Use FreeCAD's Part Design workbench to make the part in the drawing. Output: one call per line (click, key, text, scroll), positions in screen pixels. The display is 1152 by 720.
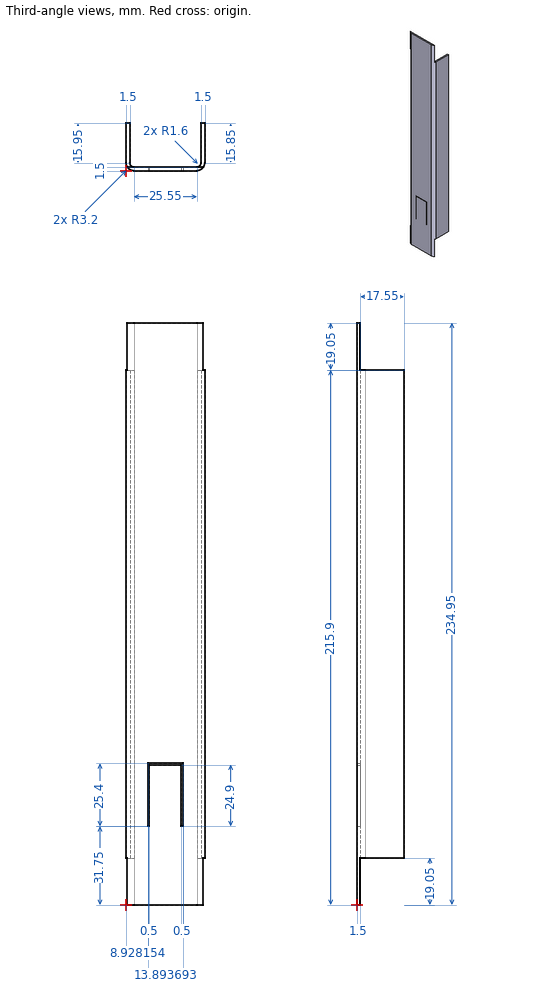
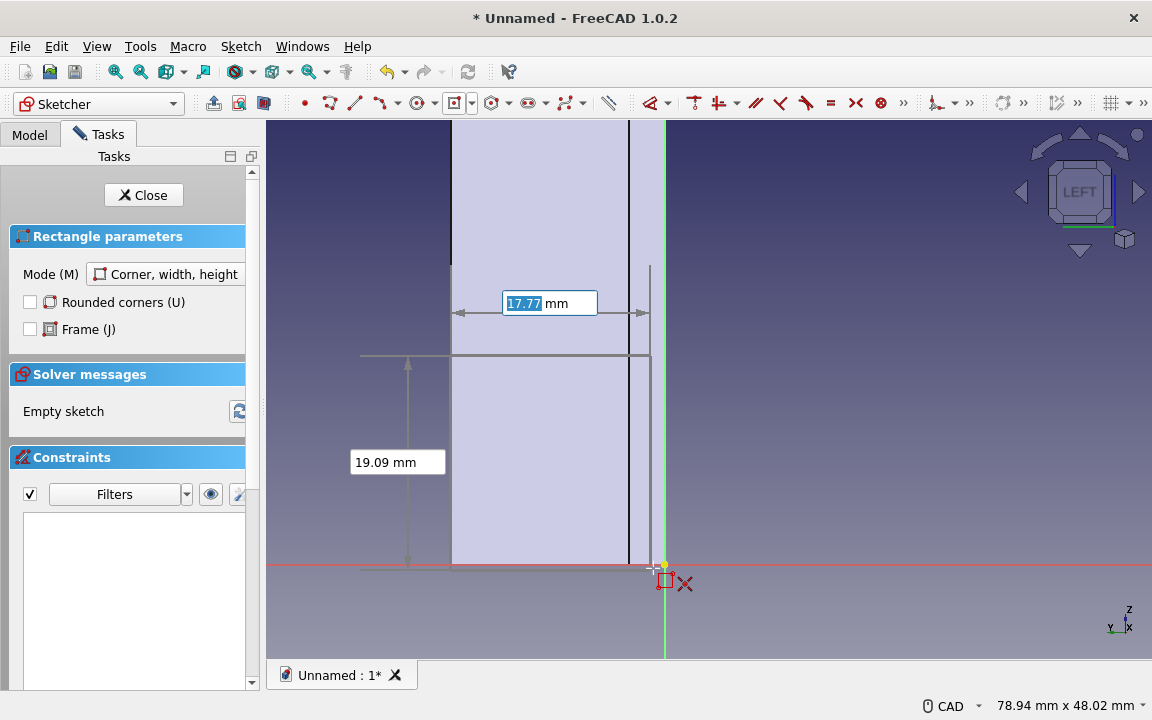
click(648, 565)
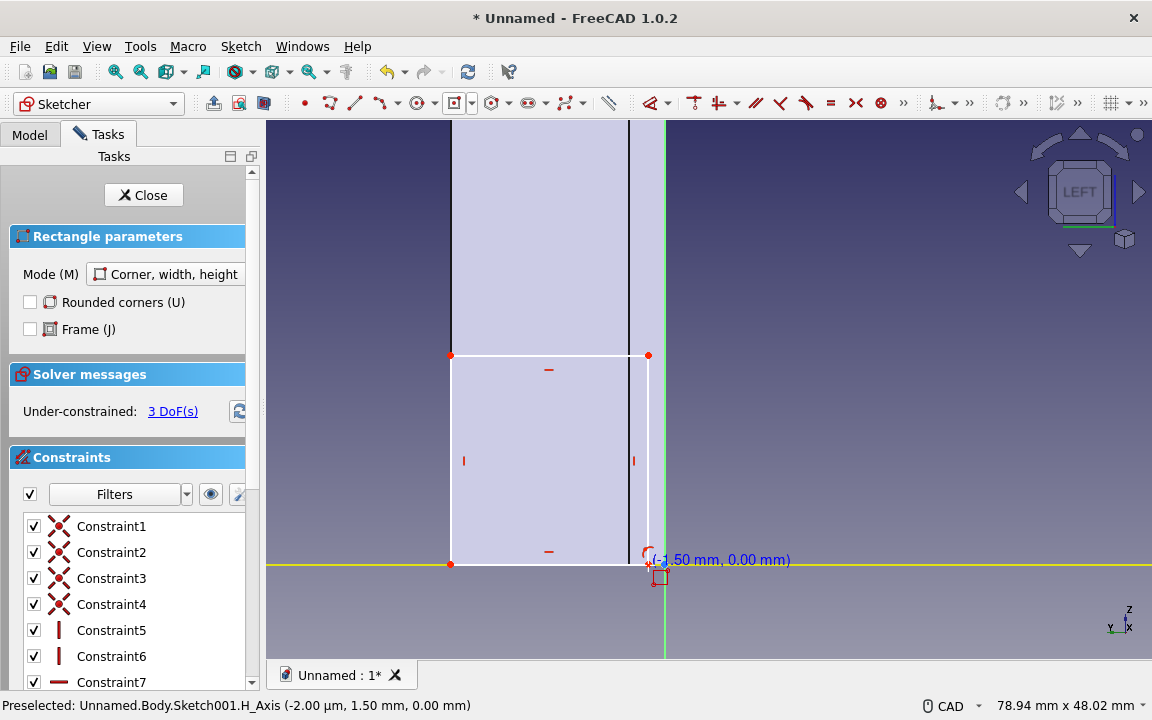
scroll(653, 568, down, 10)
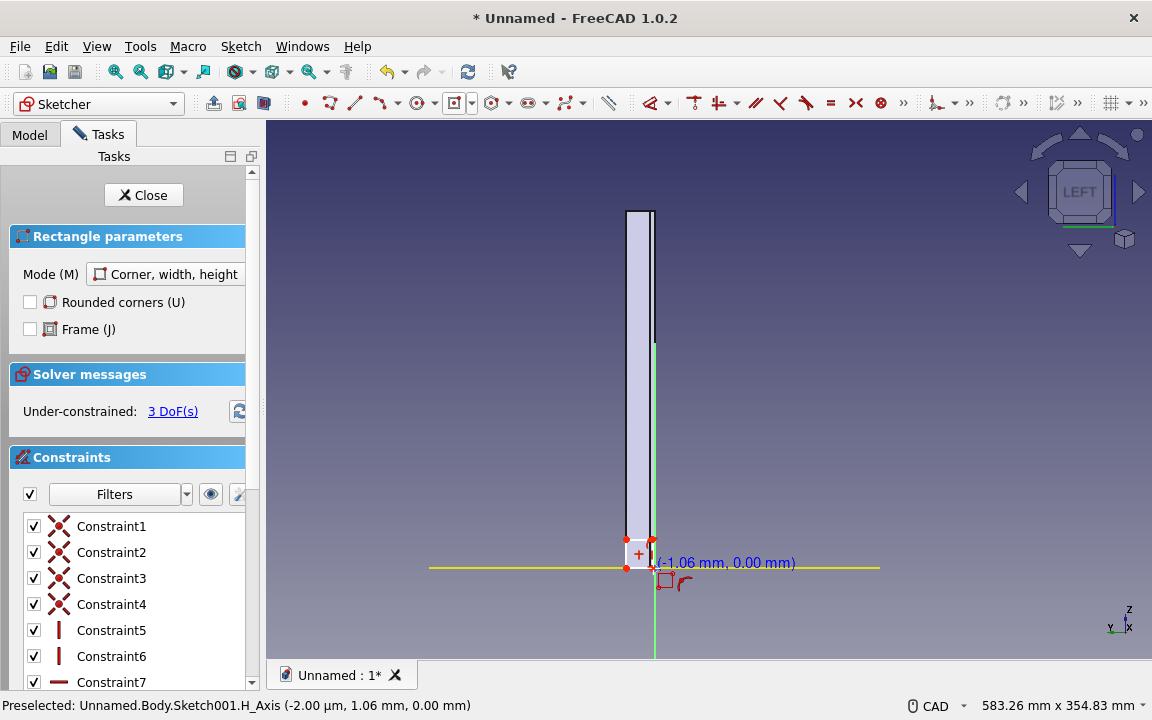
click(626, 211)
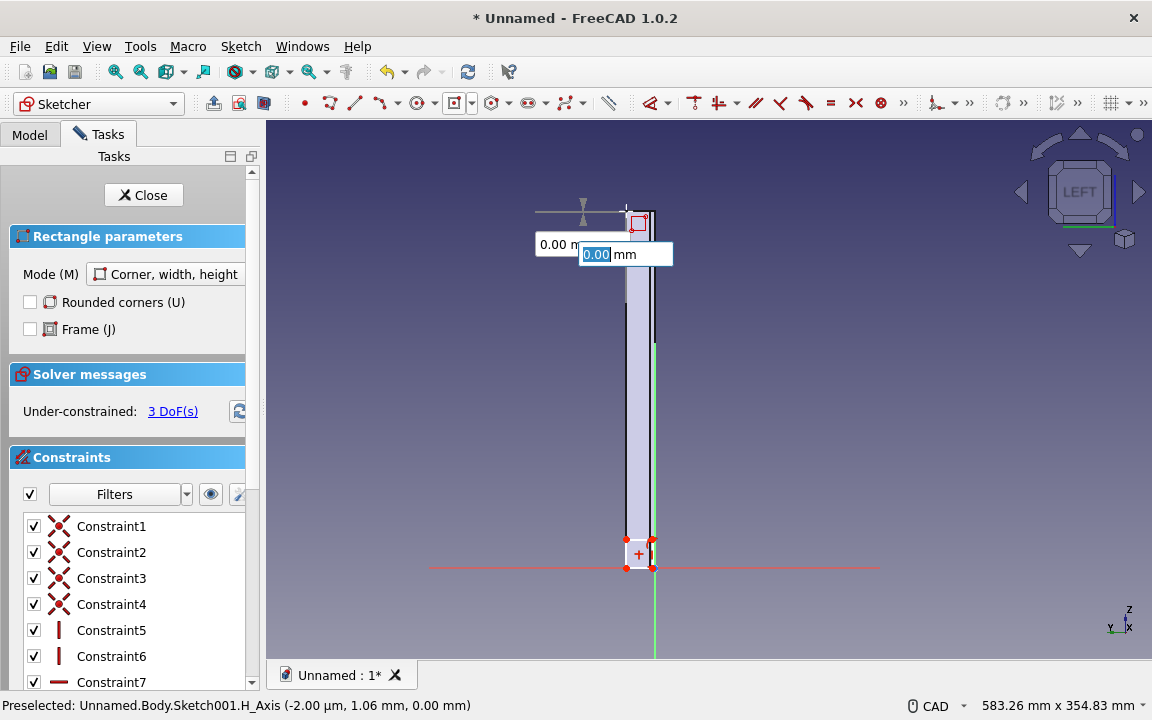
scroll(653, 240, up, 10)
move(648, 241)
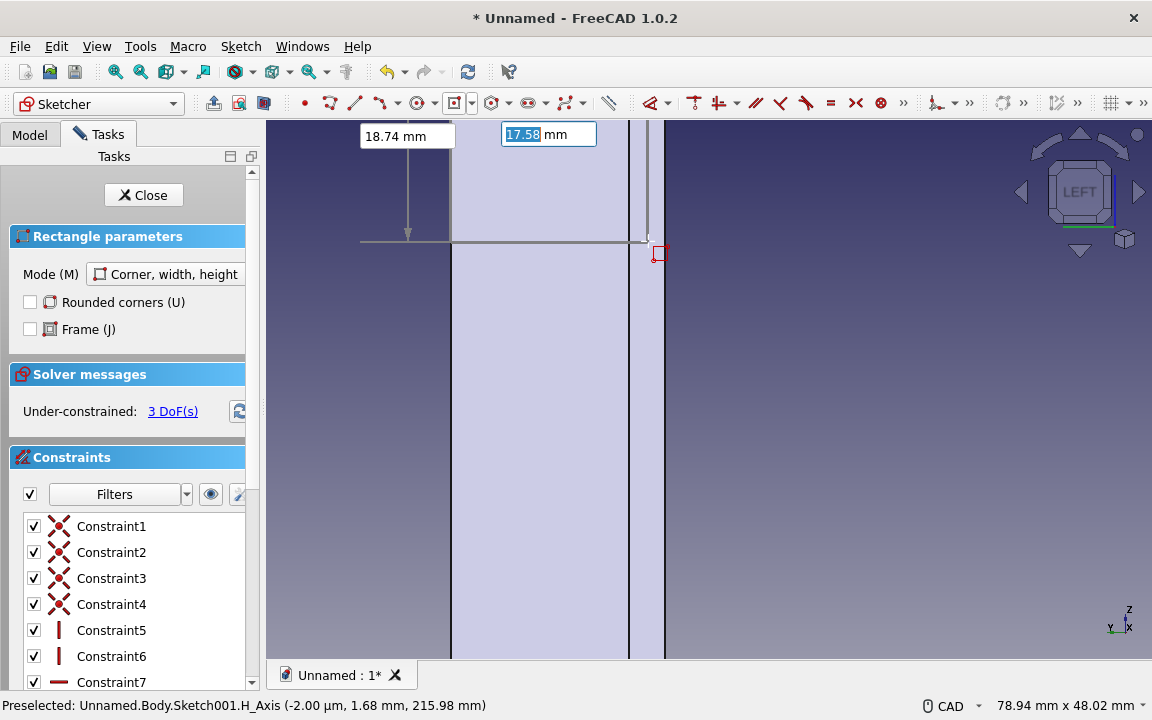
text(17.55)
key(Tab)
text(19.05)
key(Return)
key(Escape)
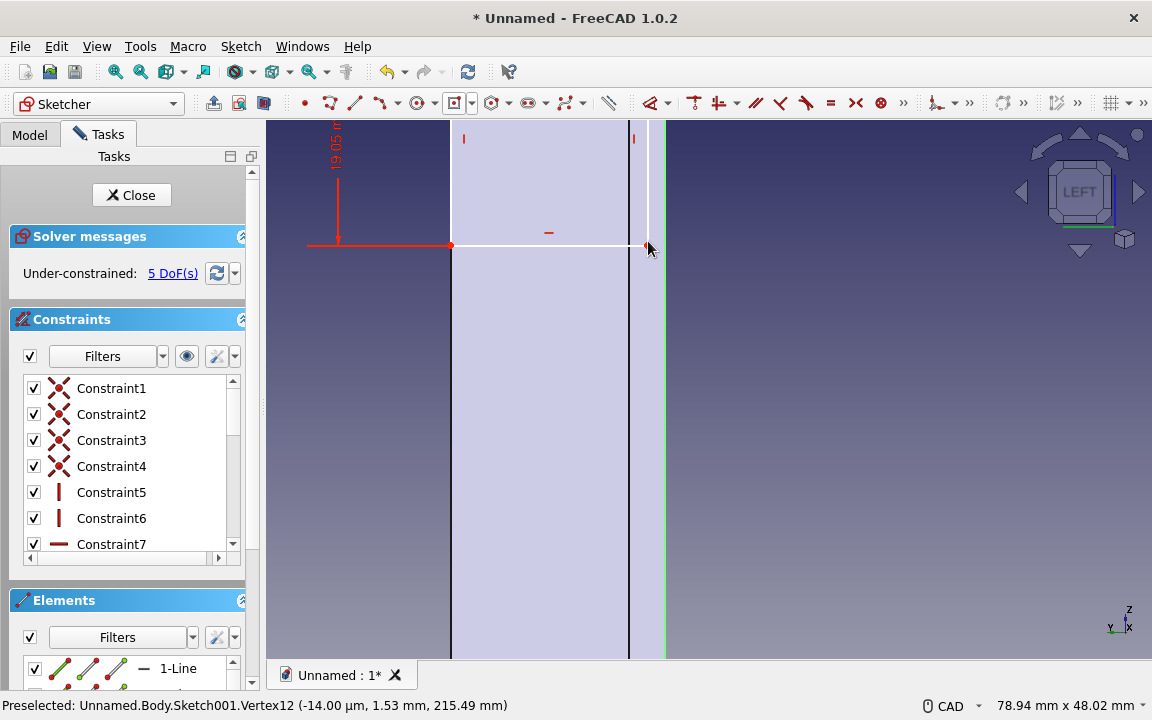
click(650, 104)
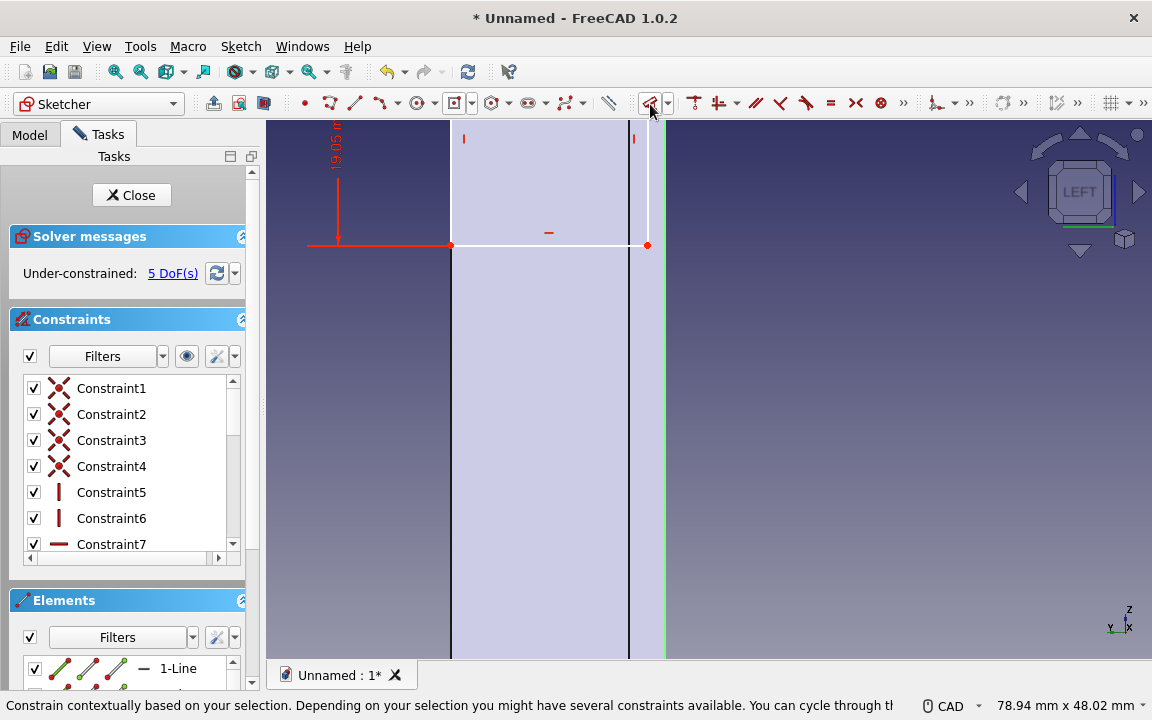
scroll(653, 240, down, 10)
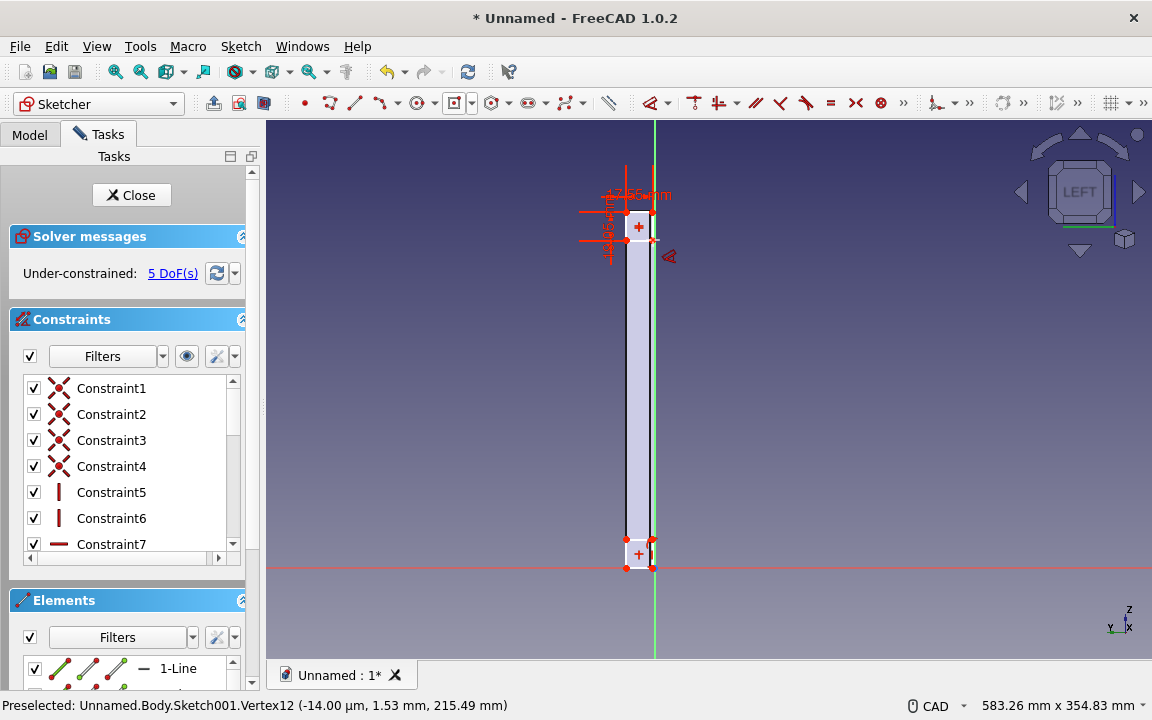
scroll(653, 568, up, 15)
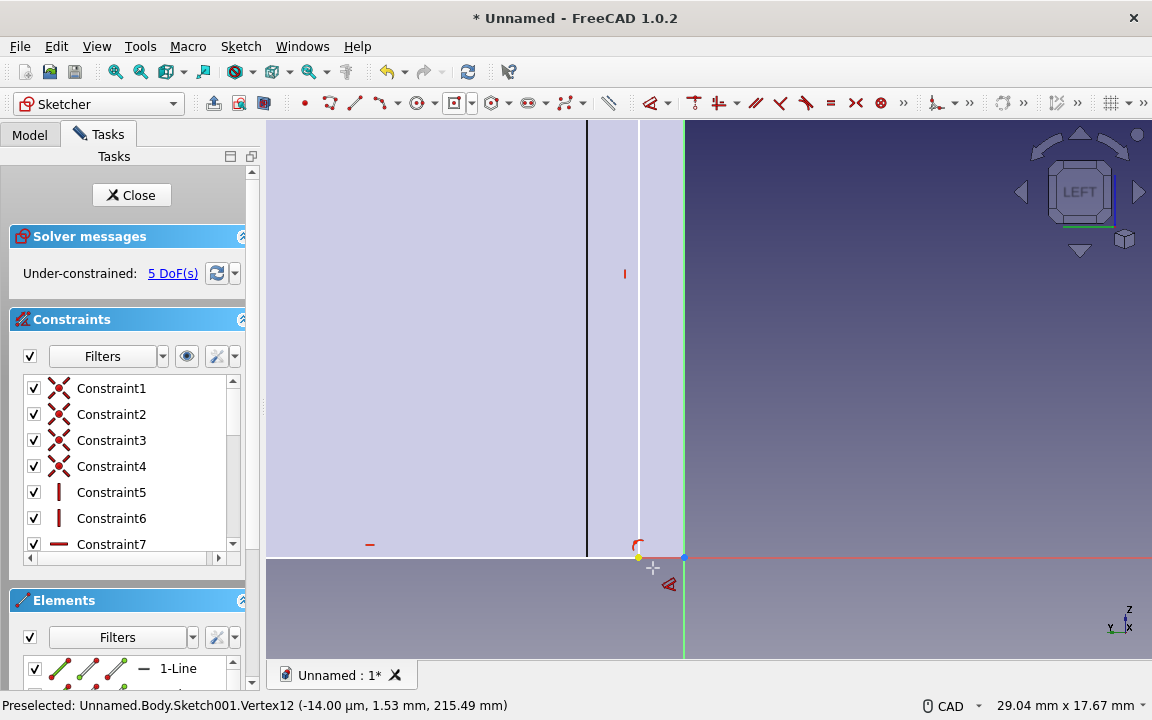
click(639, 558)
click(662, 592)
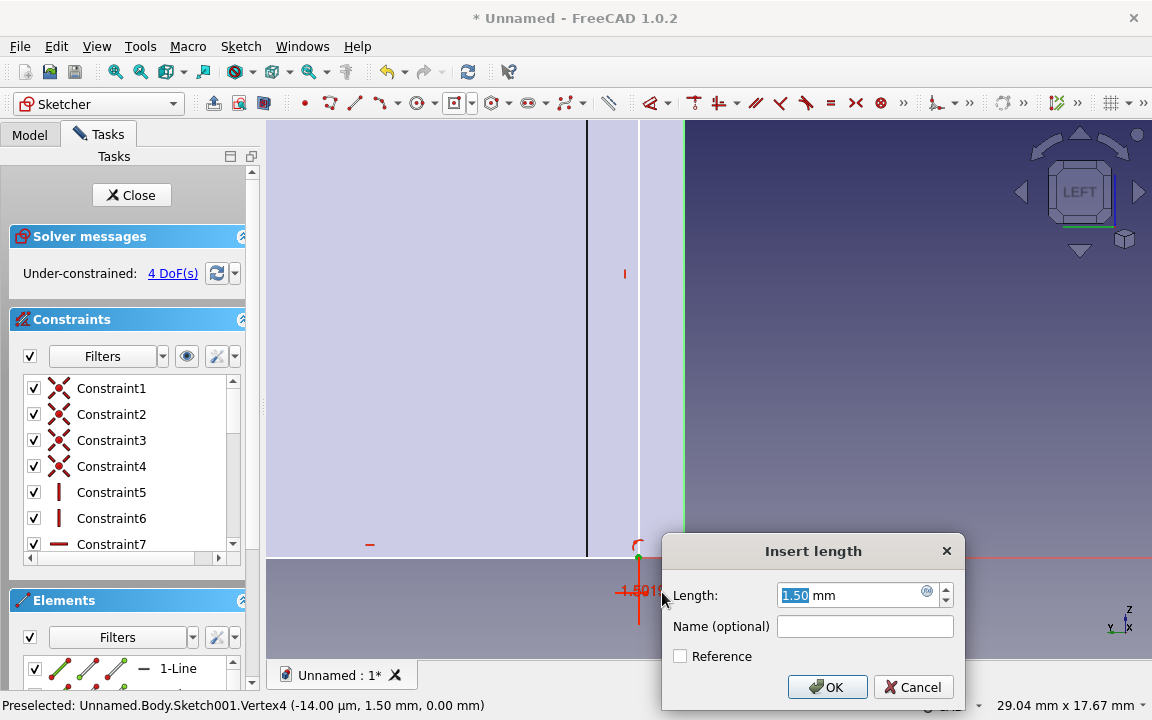
text(1.5)
key(Return)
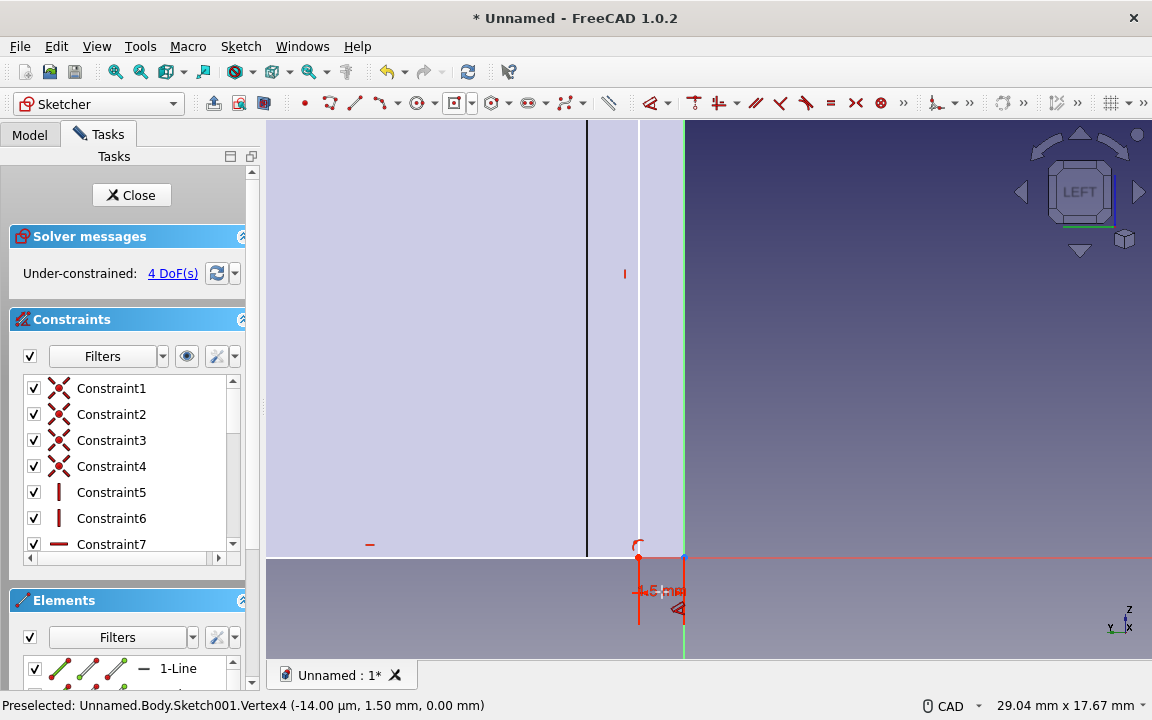
scroll(653, 568, down, 15)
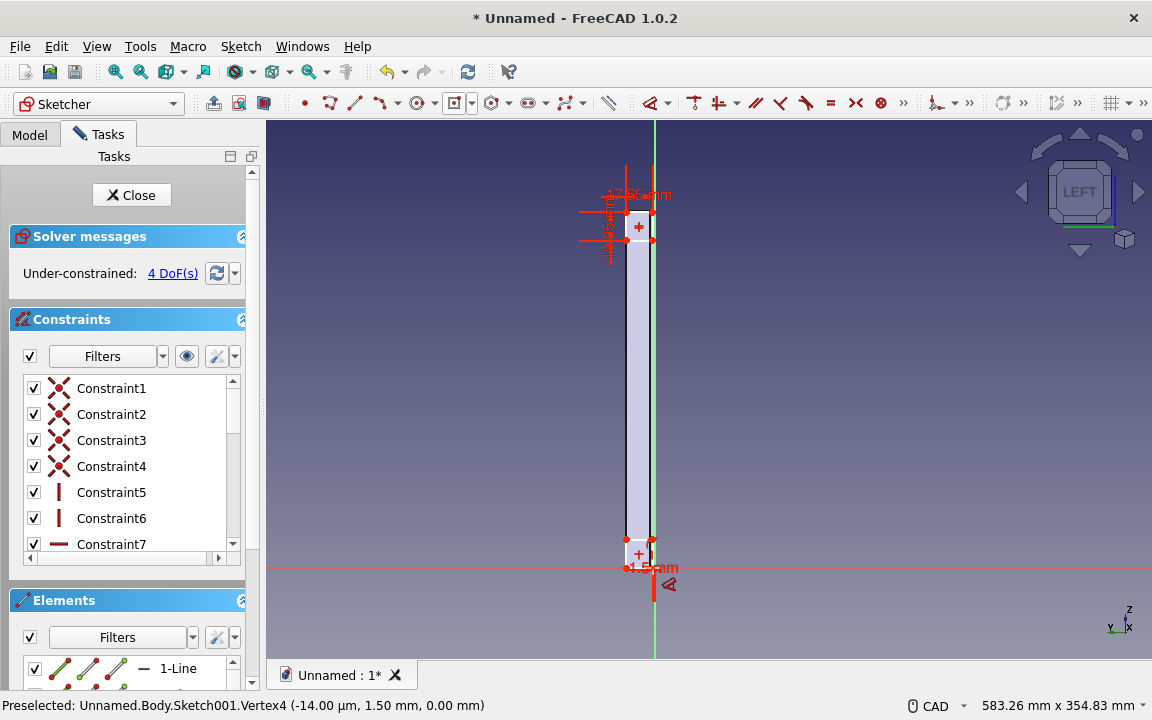
scroll(653, 241, up, 15)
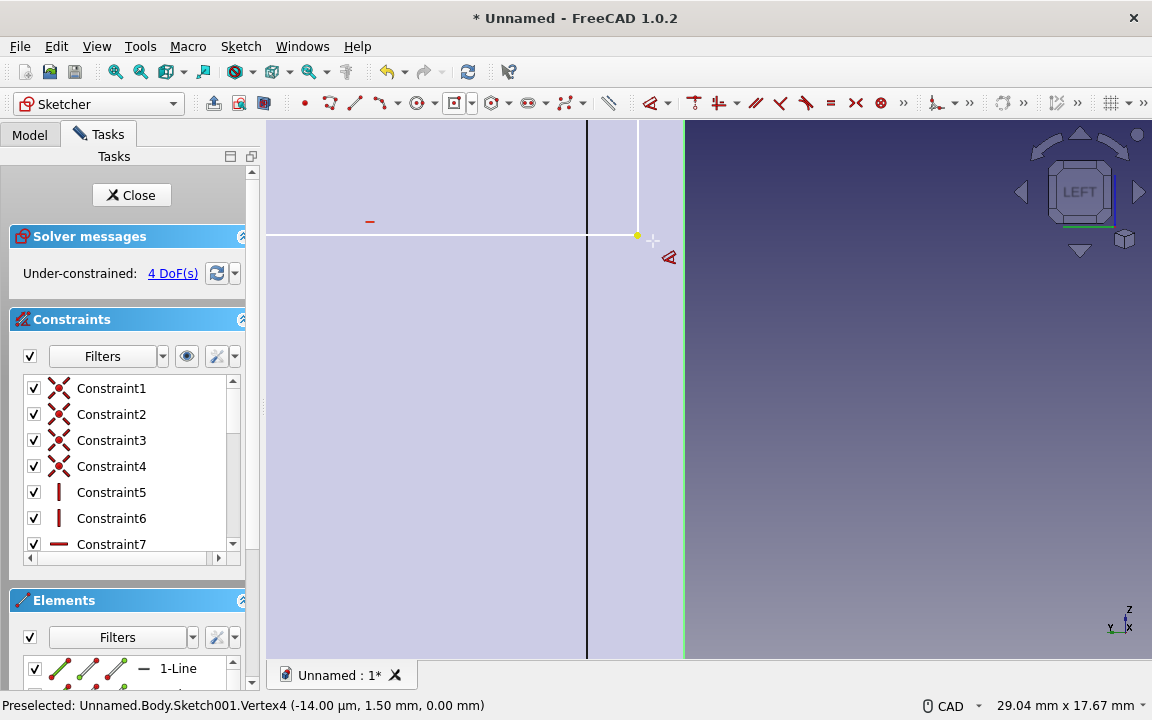
click(638, 235)
click(661, 201)